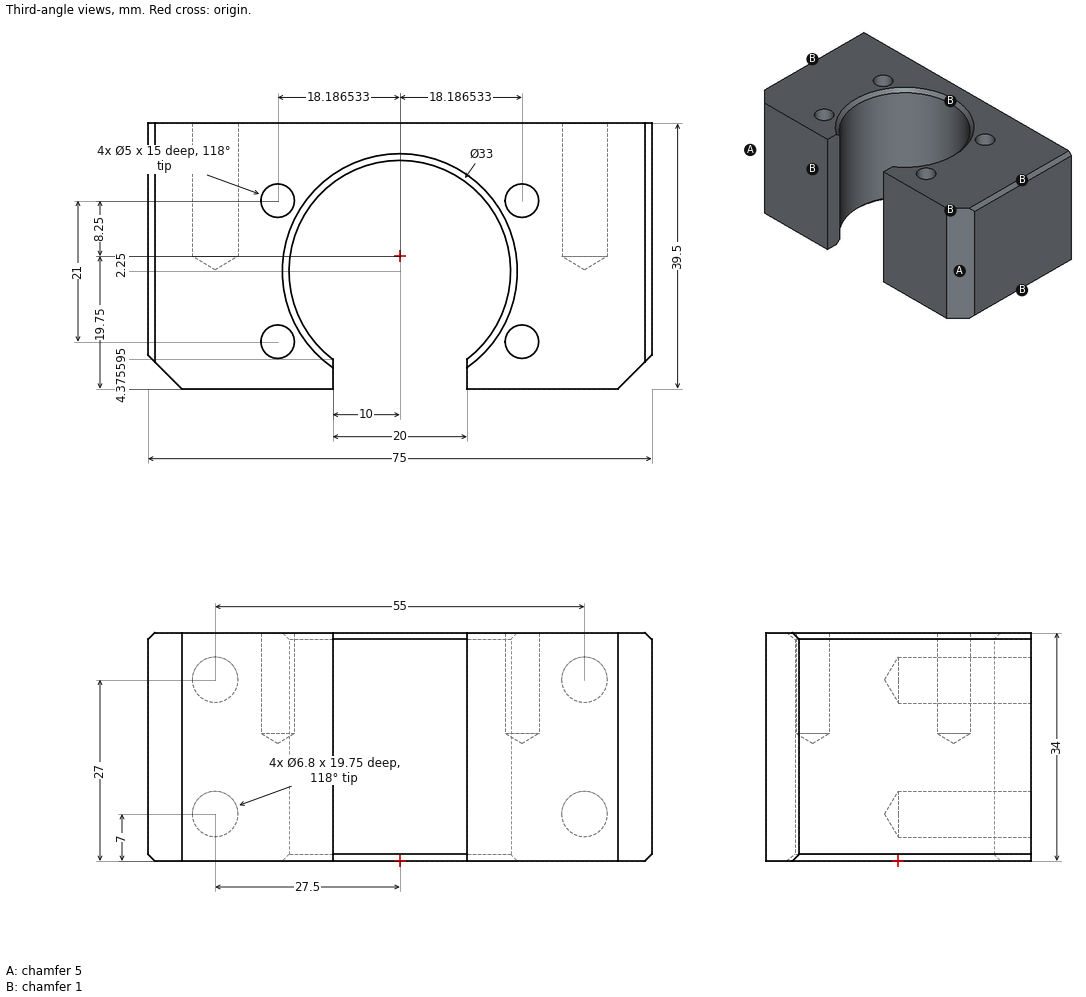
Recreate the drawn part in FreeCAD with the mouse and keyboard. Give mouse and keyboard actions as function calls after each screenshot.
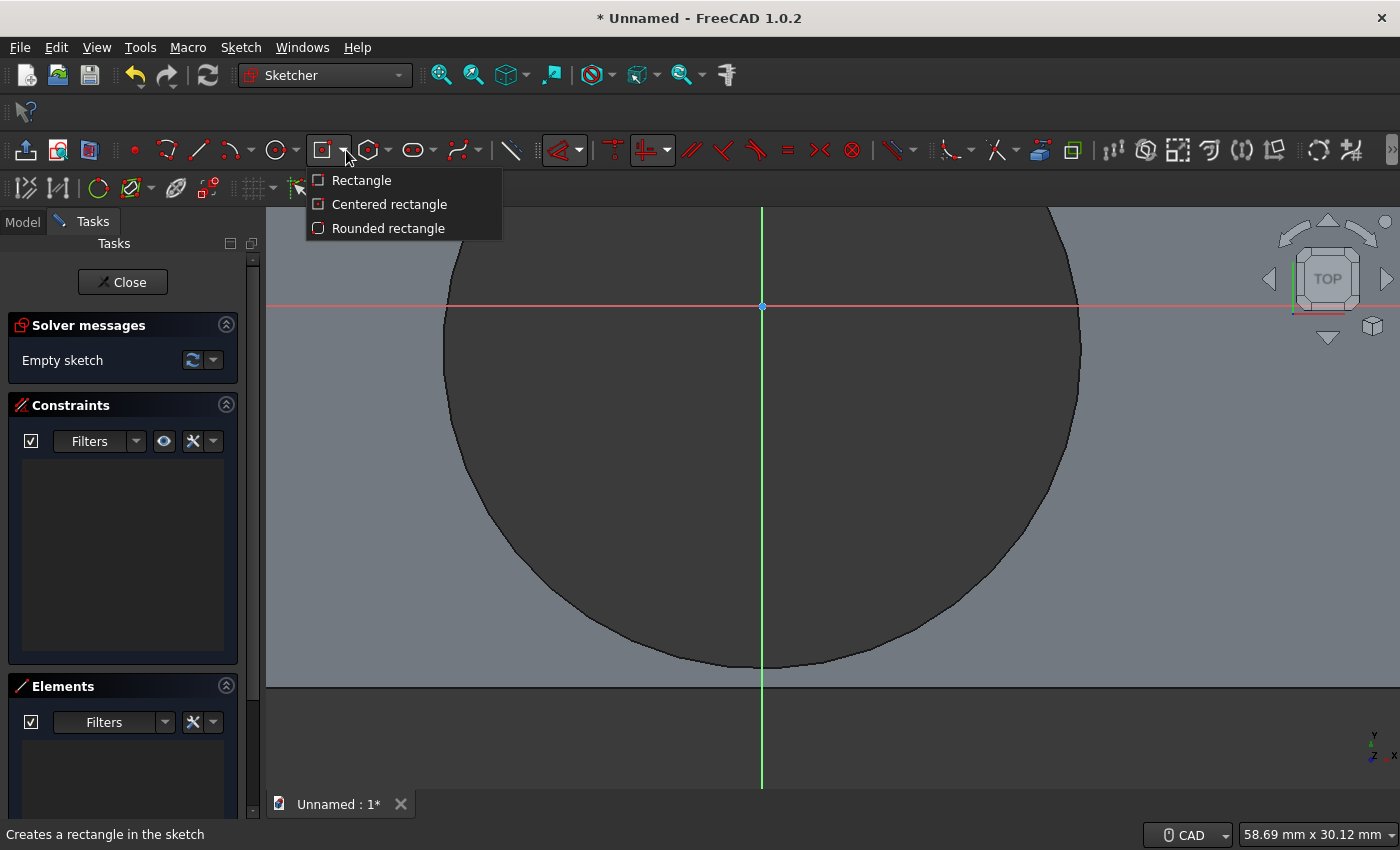
click(404, 180)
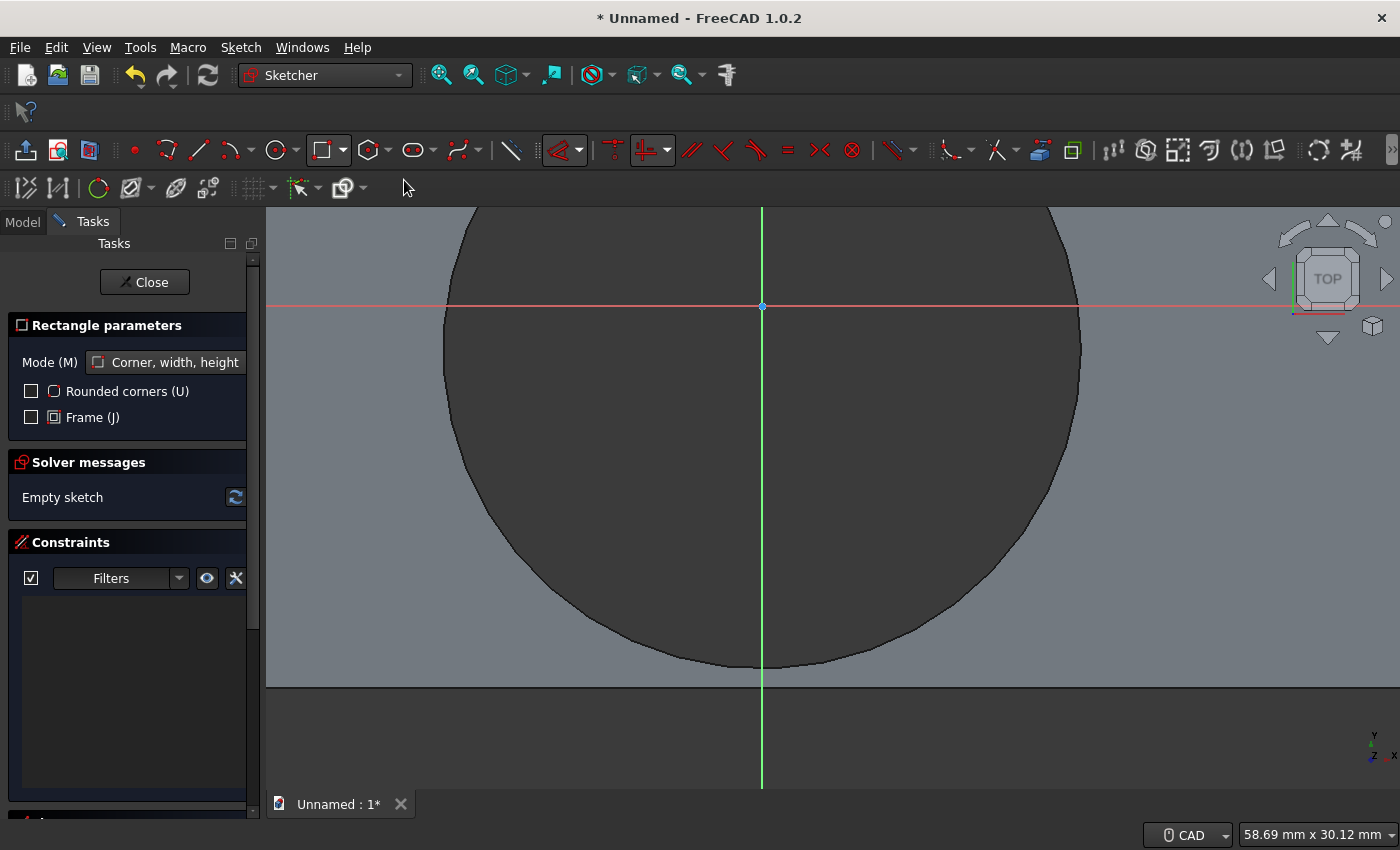
click(569, 603)
click(955, 688)
key(Escape)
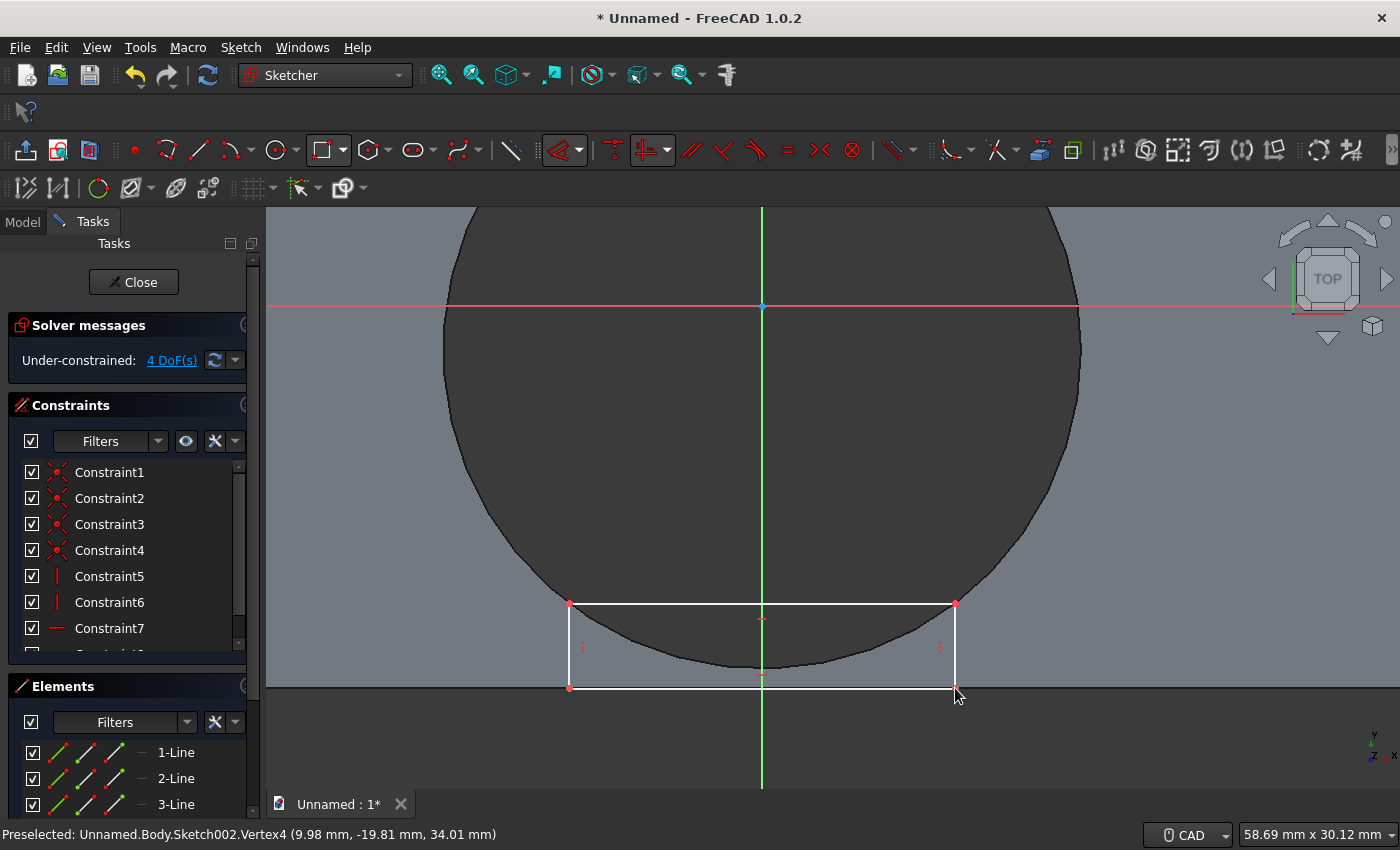
click(685, 689)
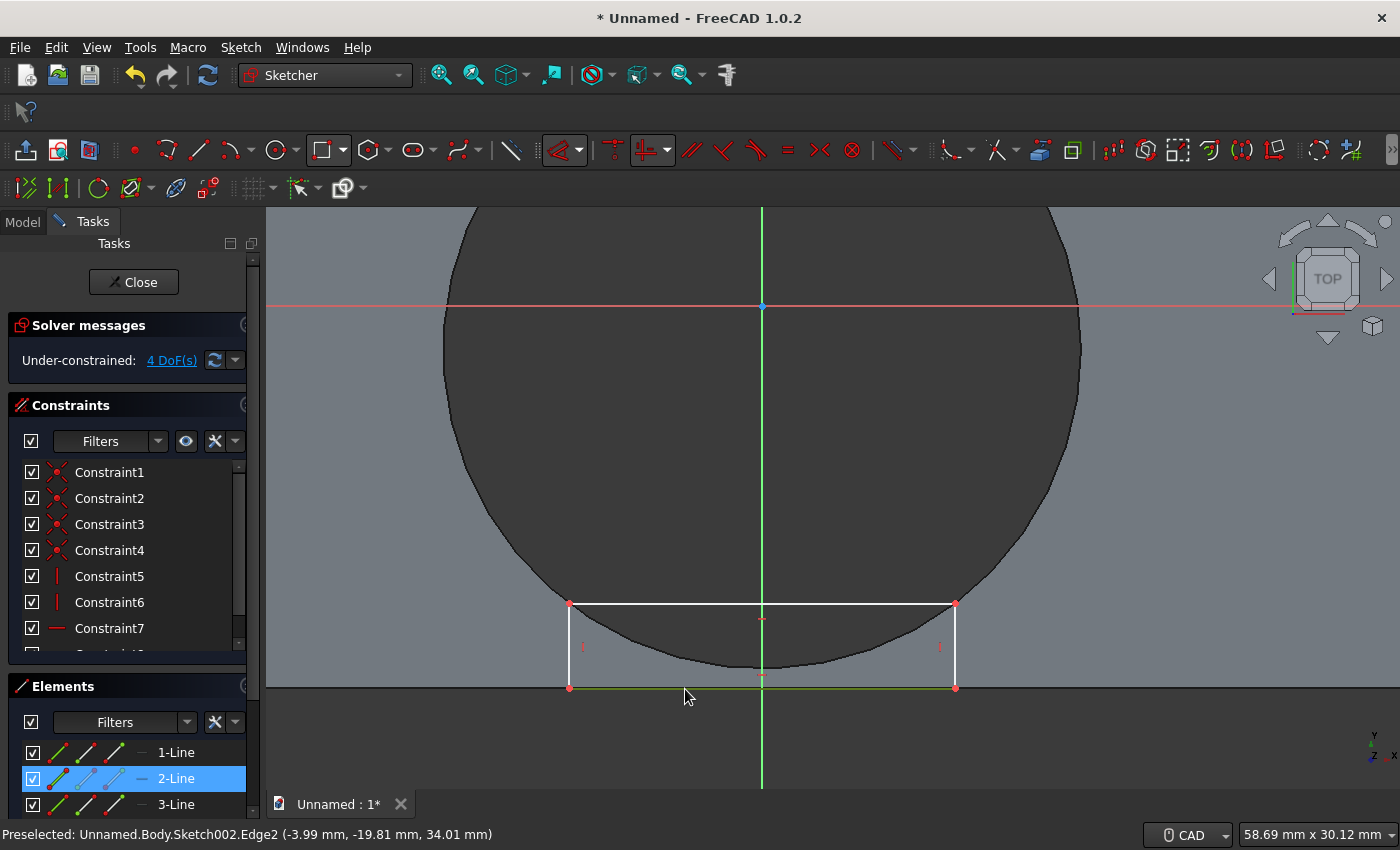
click(582, 150)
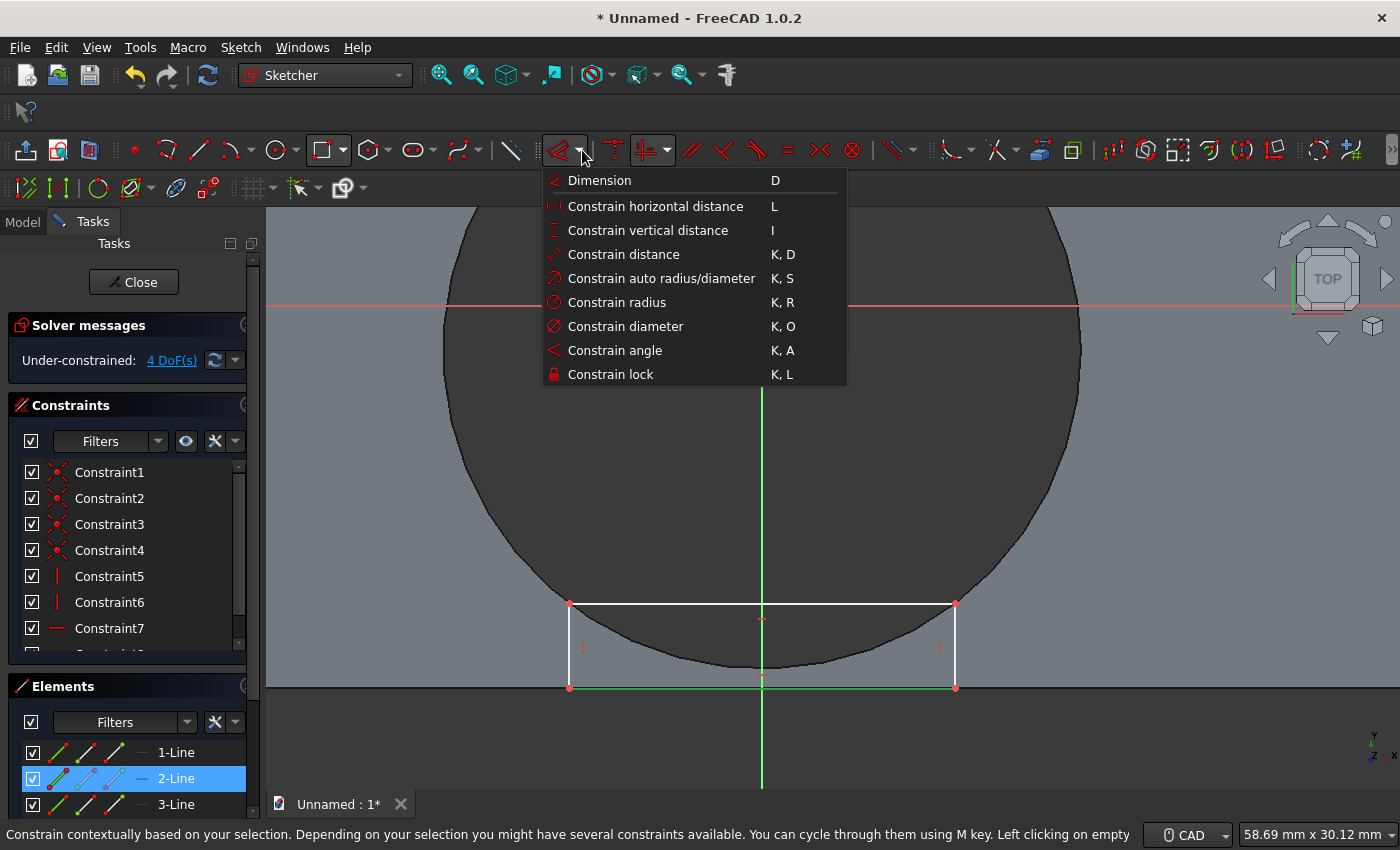
click(695, 206)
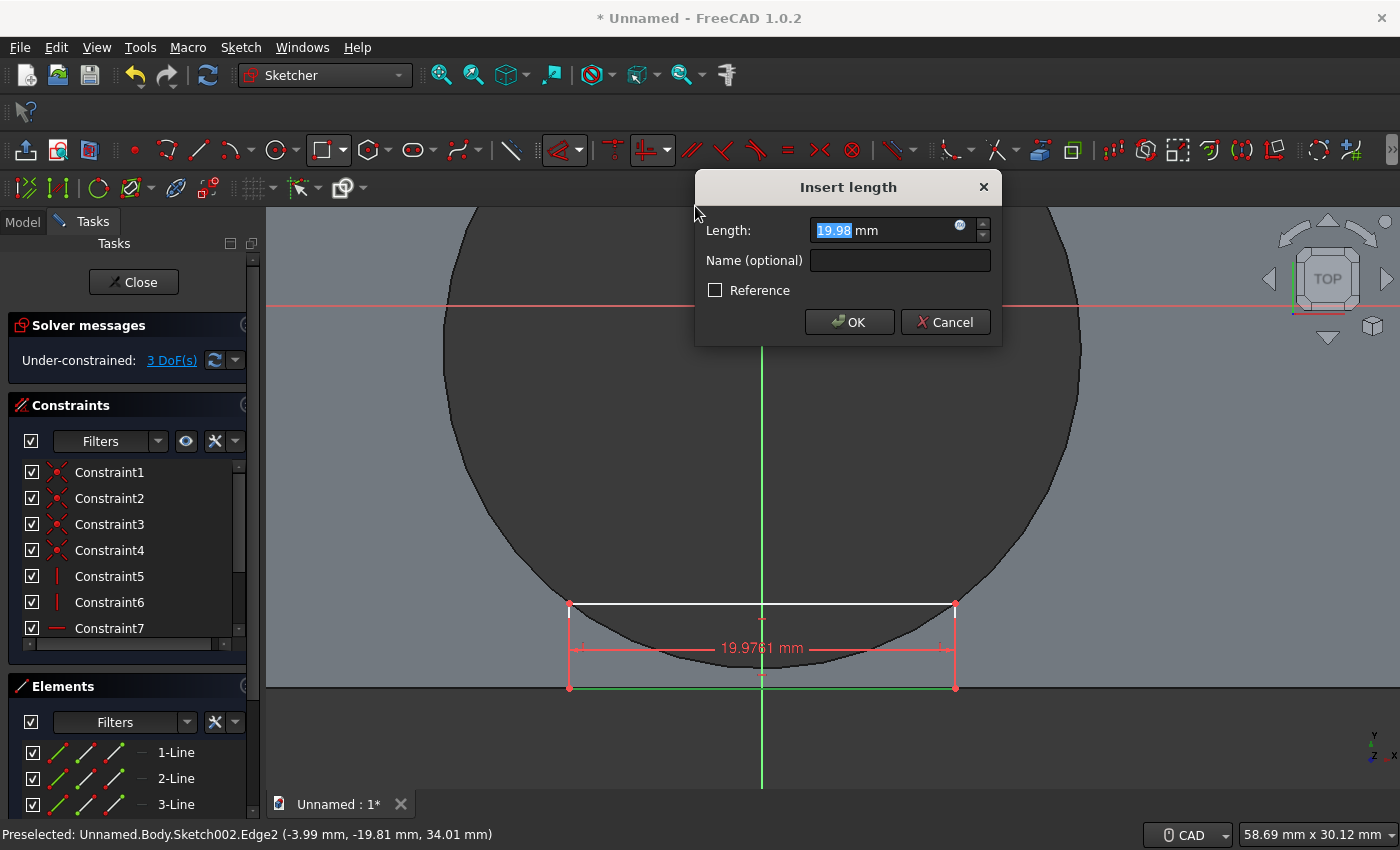
text(20)
key(Return)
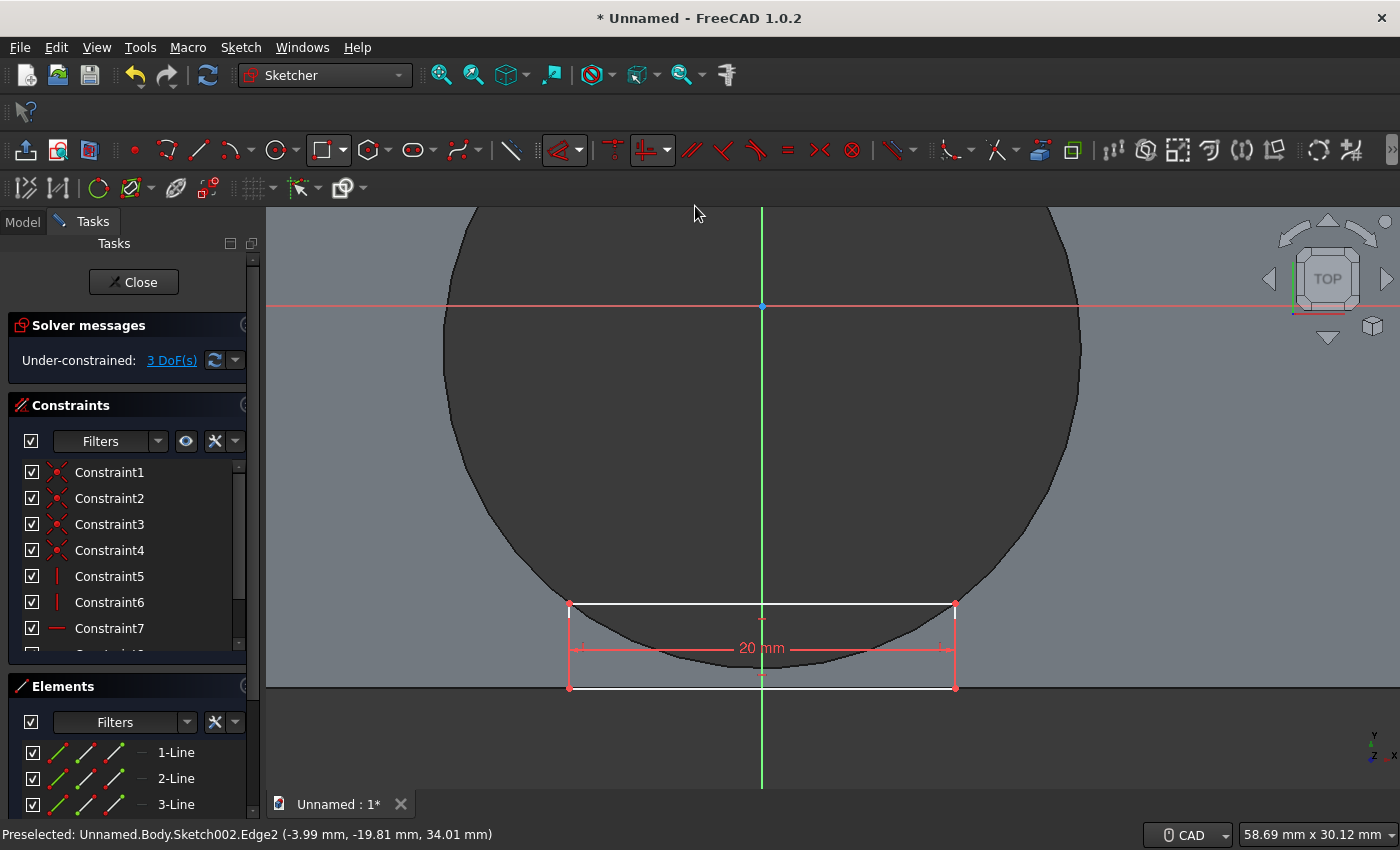
click(569, 604)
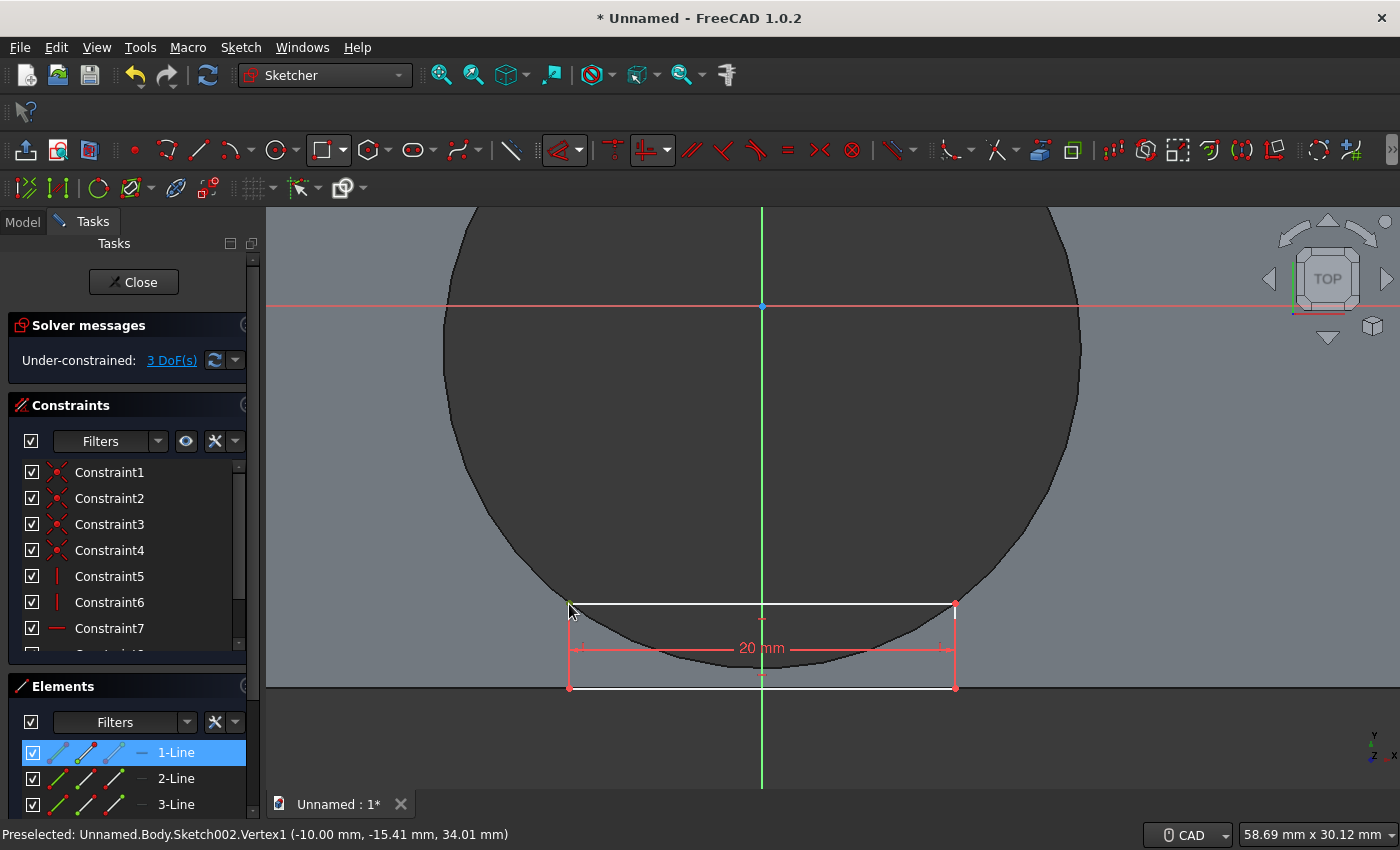
key(l)